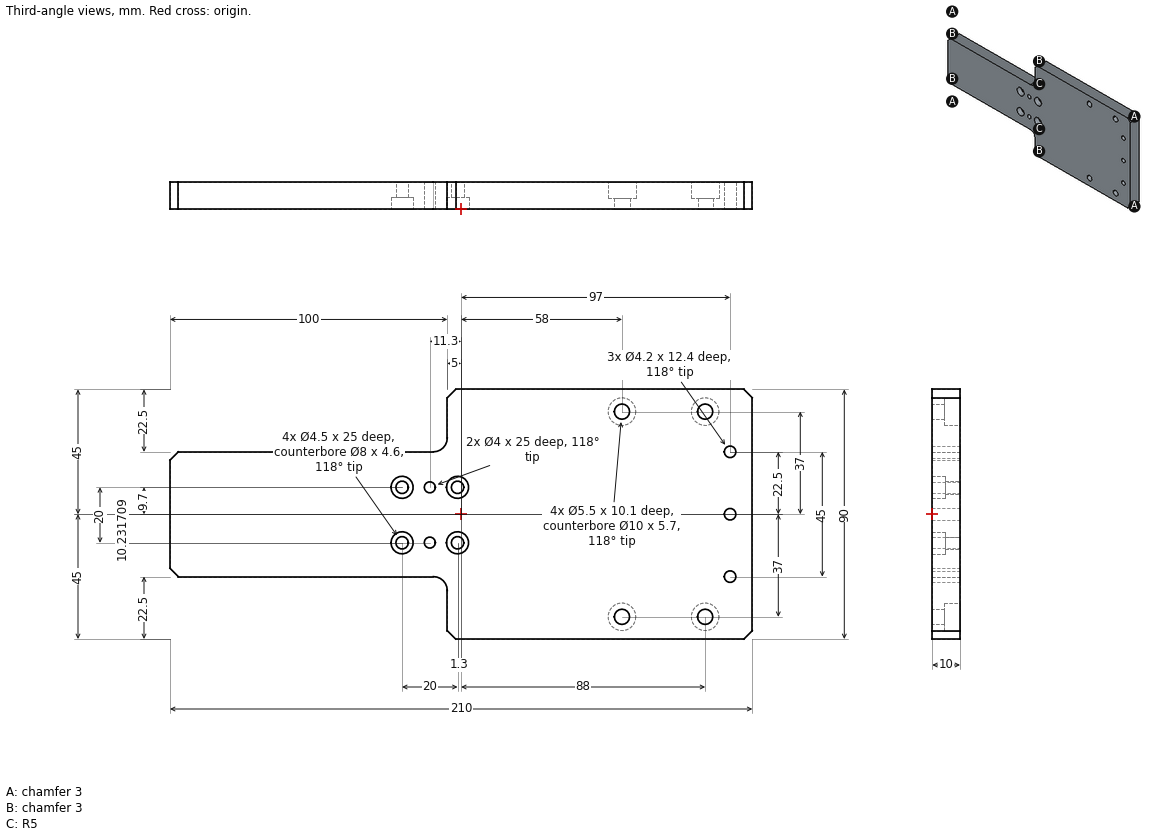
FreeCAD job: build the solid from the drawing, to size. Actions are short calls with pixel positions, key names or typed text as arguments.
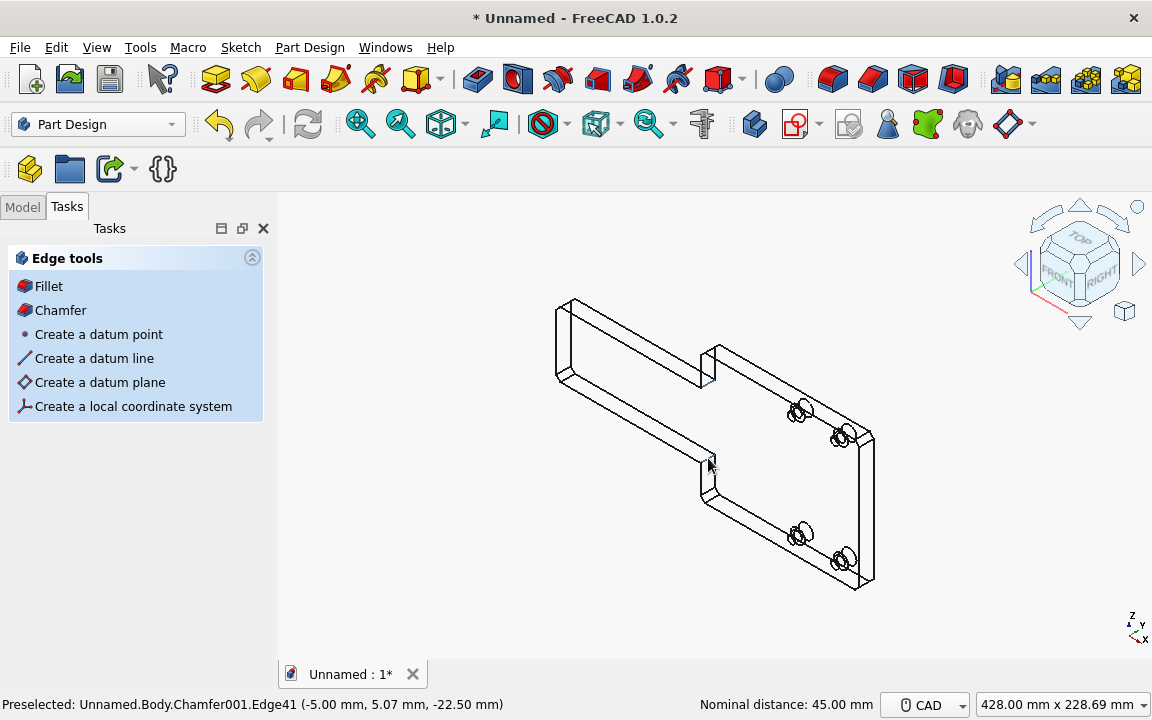
click(834, 80)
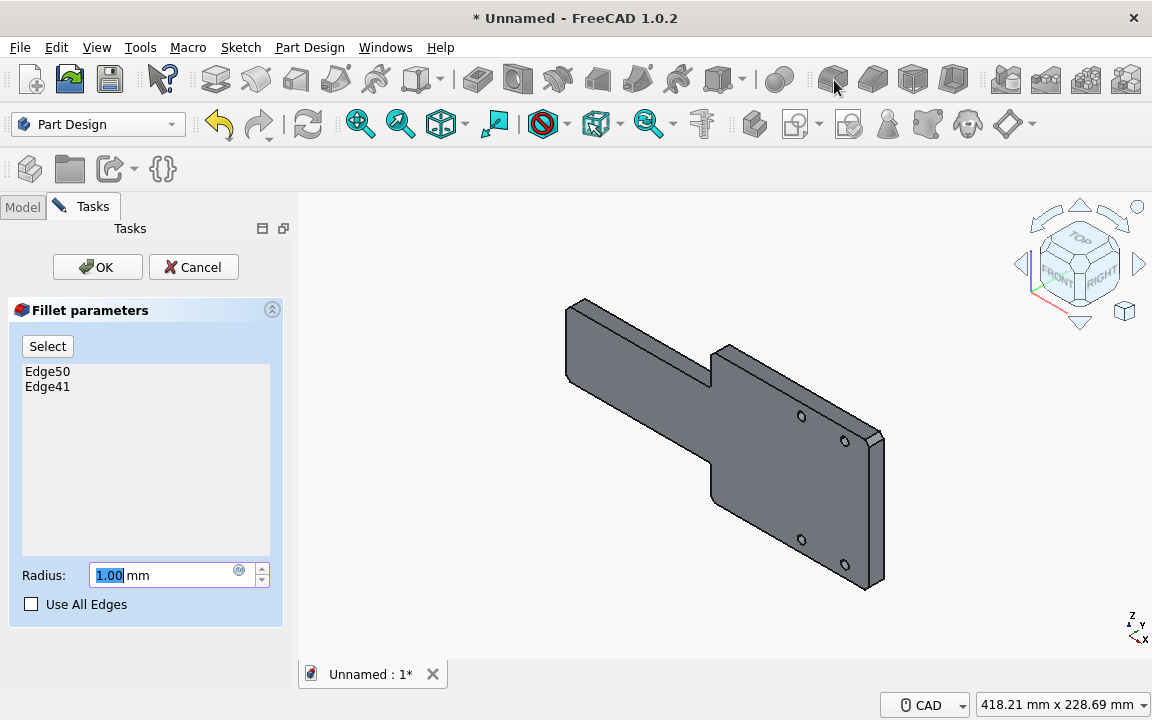
text(5)
key(Tab)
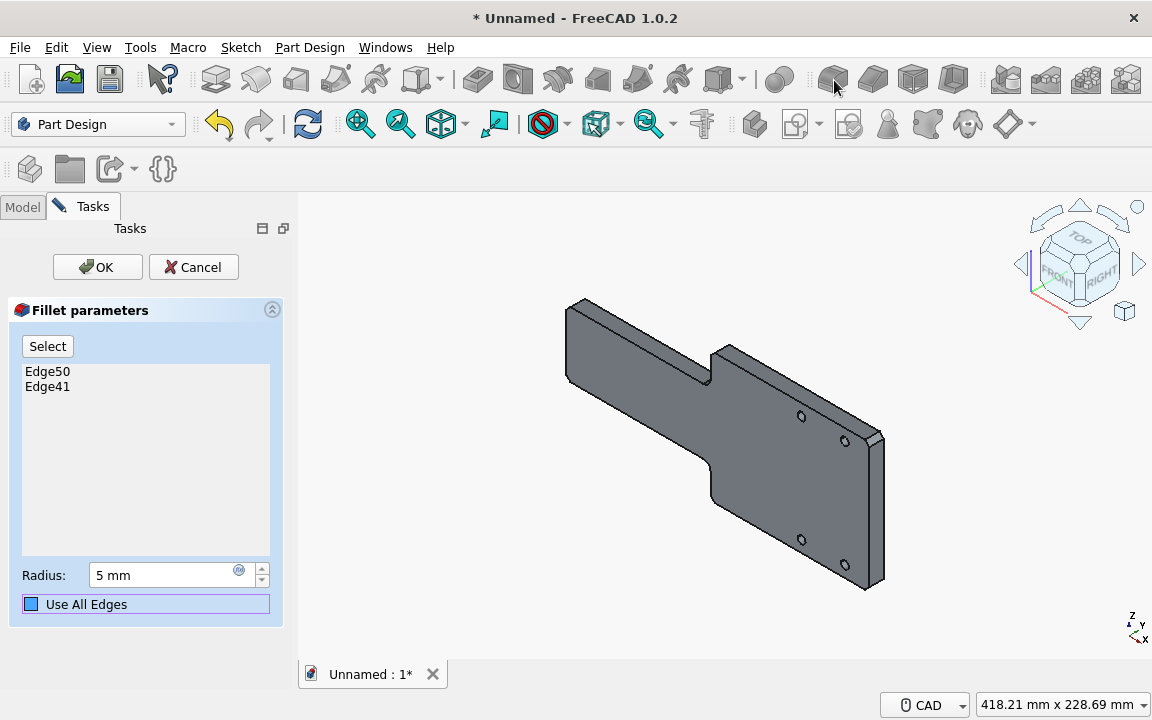
click(98, 267)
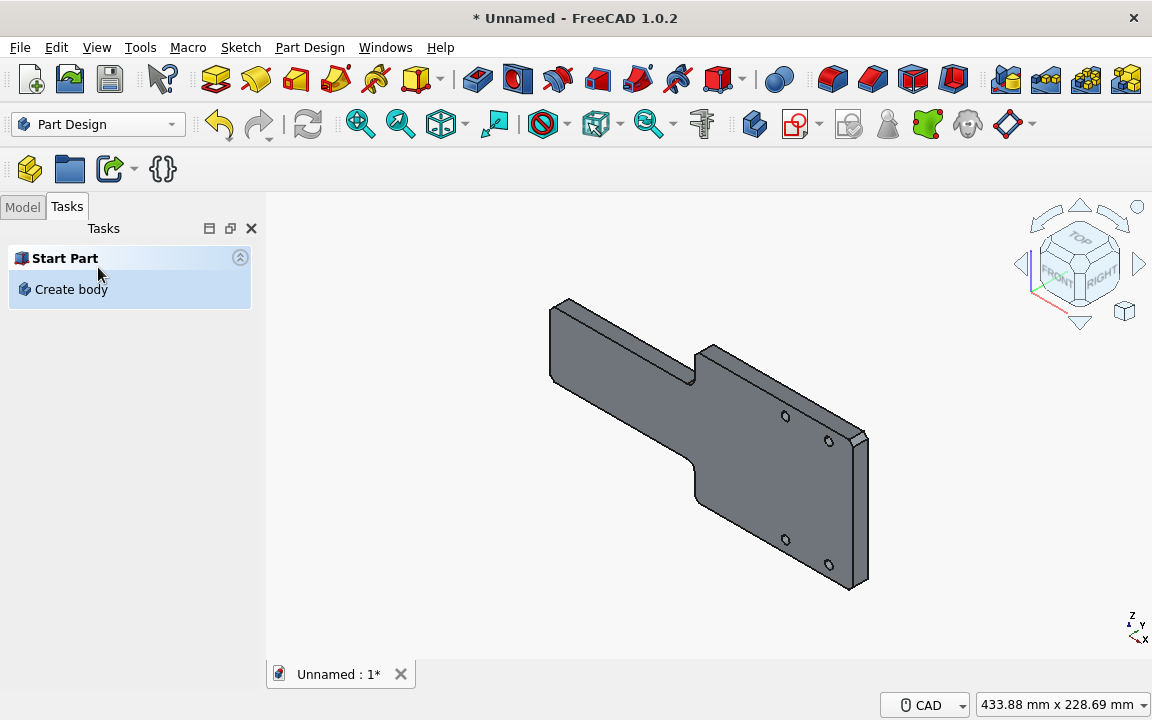
click(796, 124)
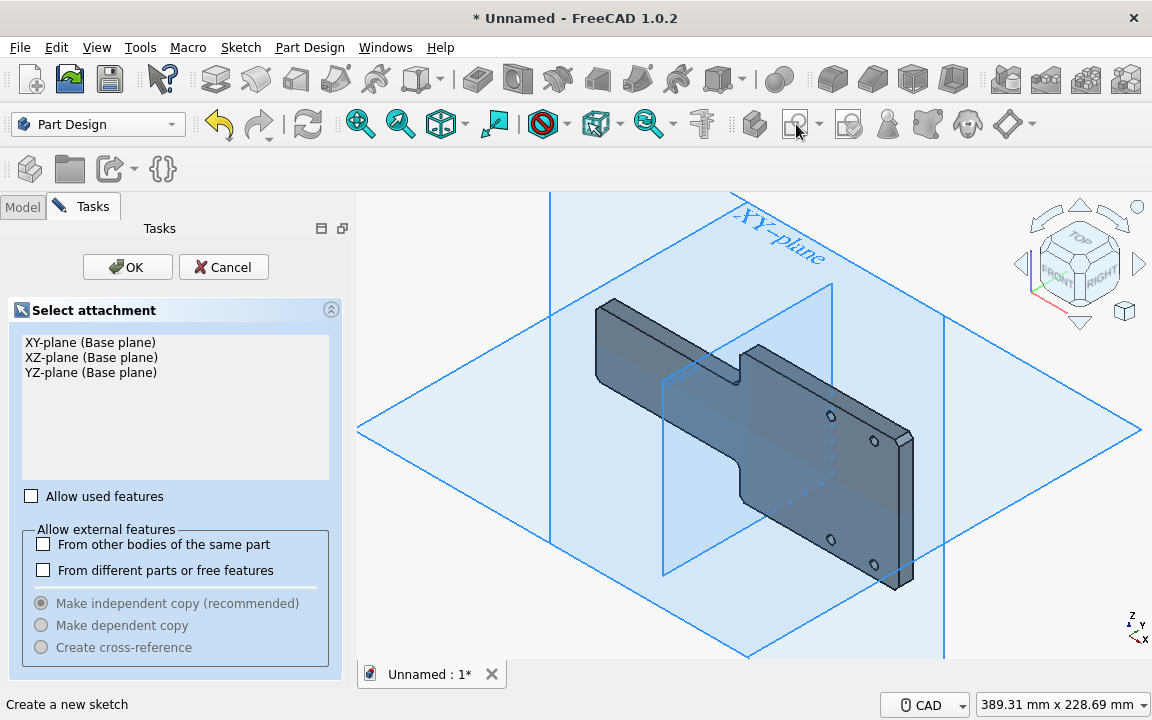
click(82, 358)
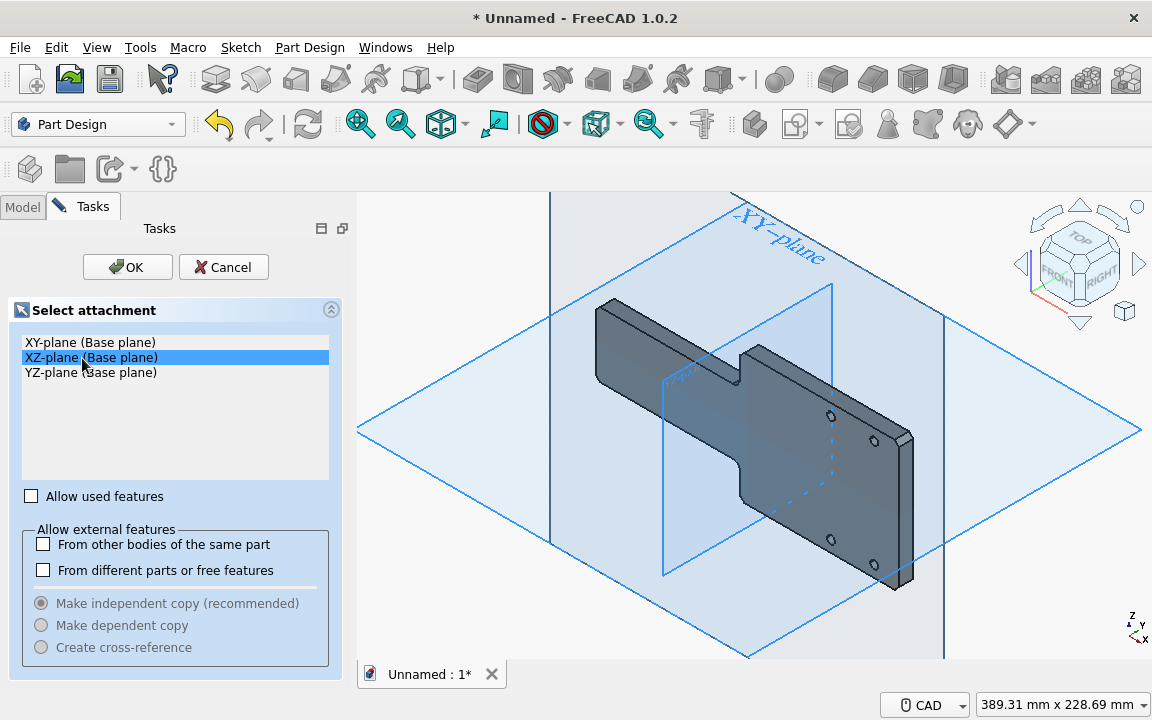
click(128, 267)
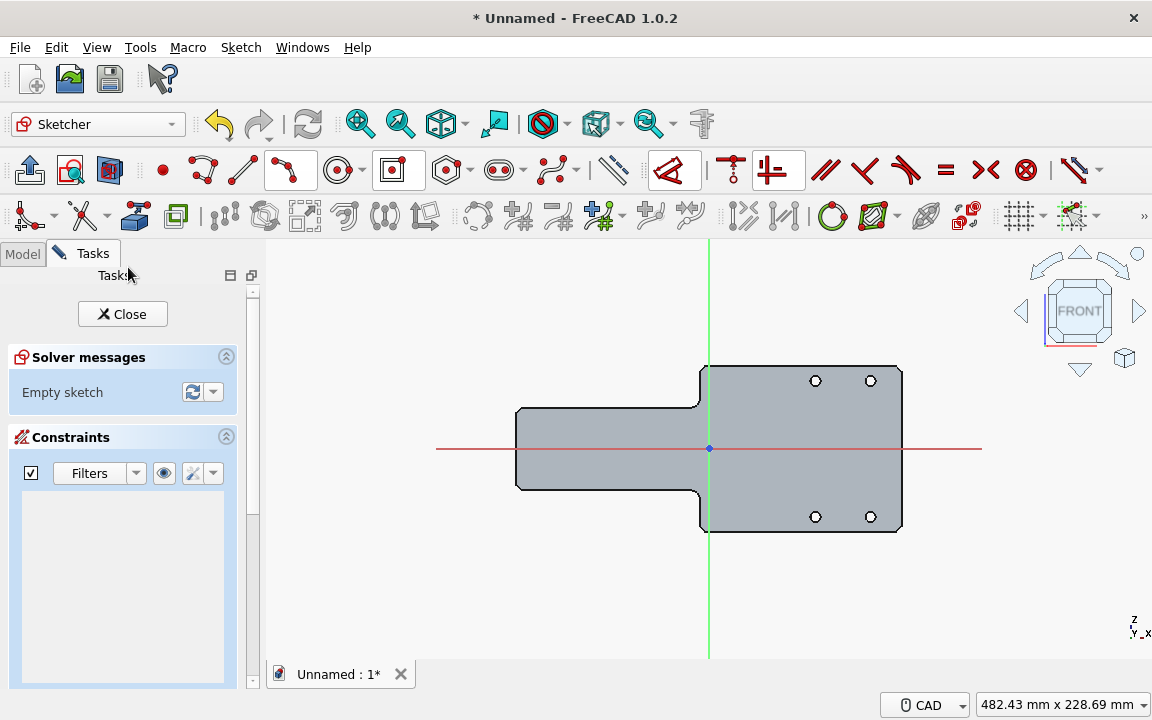
scroll(698, 450, up, 9)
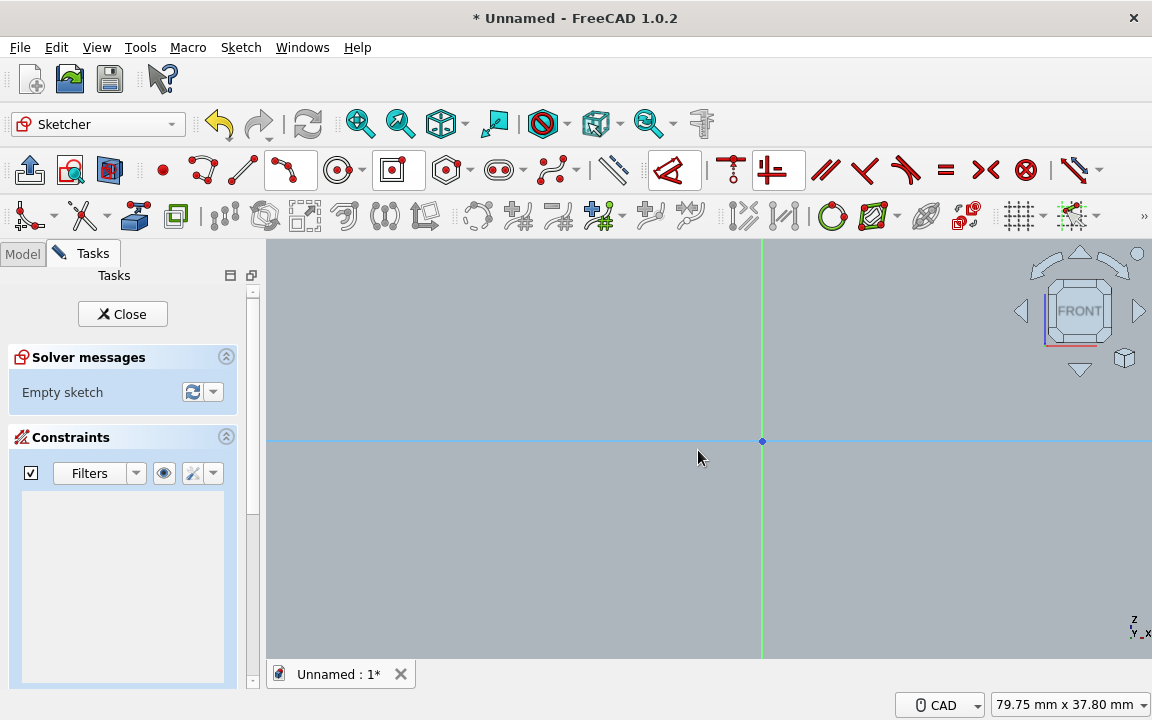
click(338, 170)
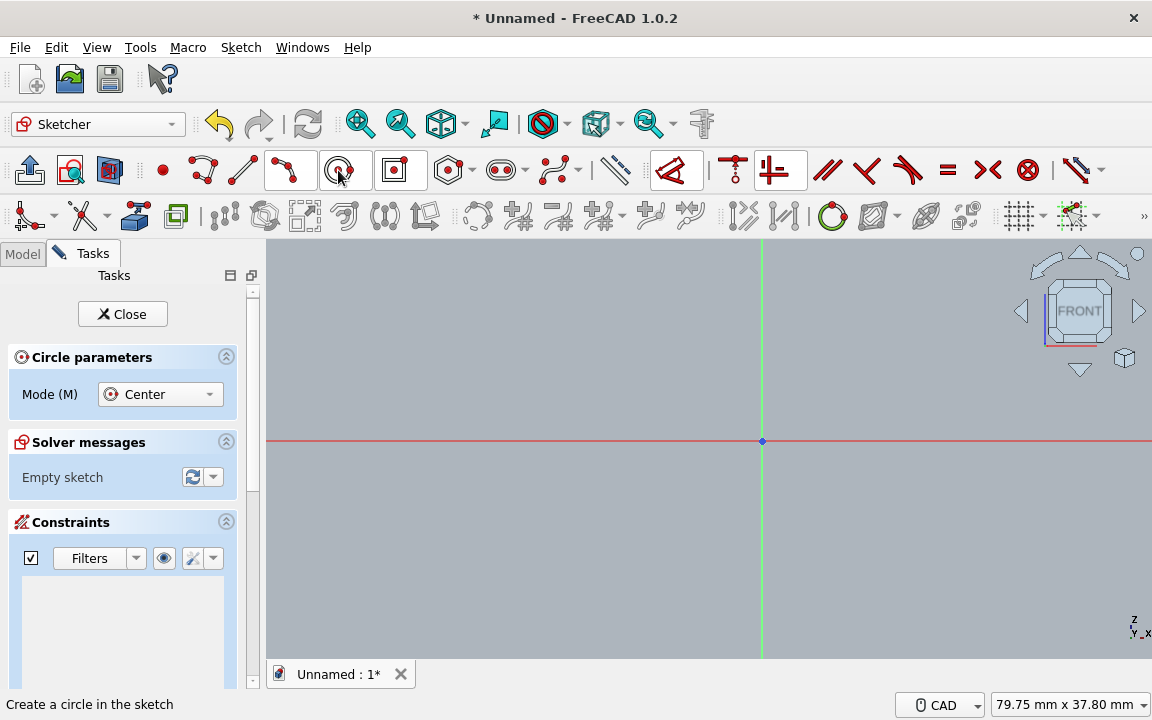
click(525, 556)
click(543, 538)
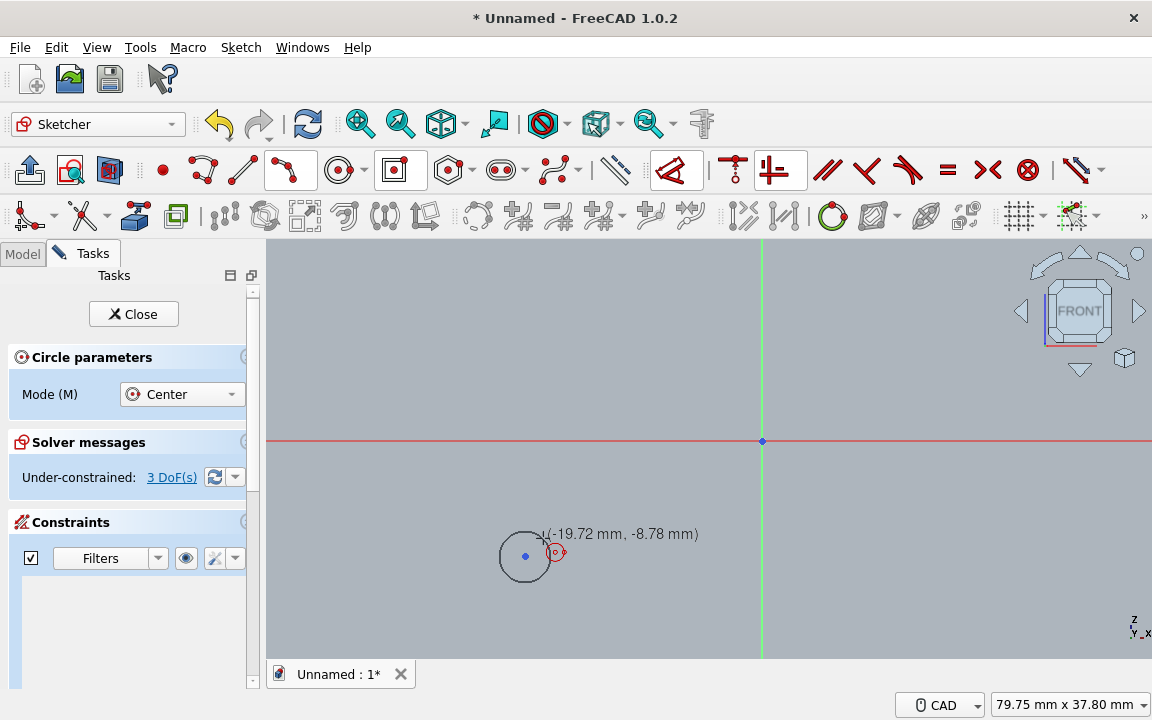
click(525, 334)
click(543, 316)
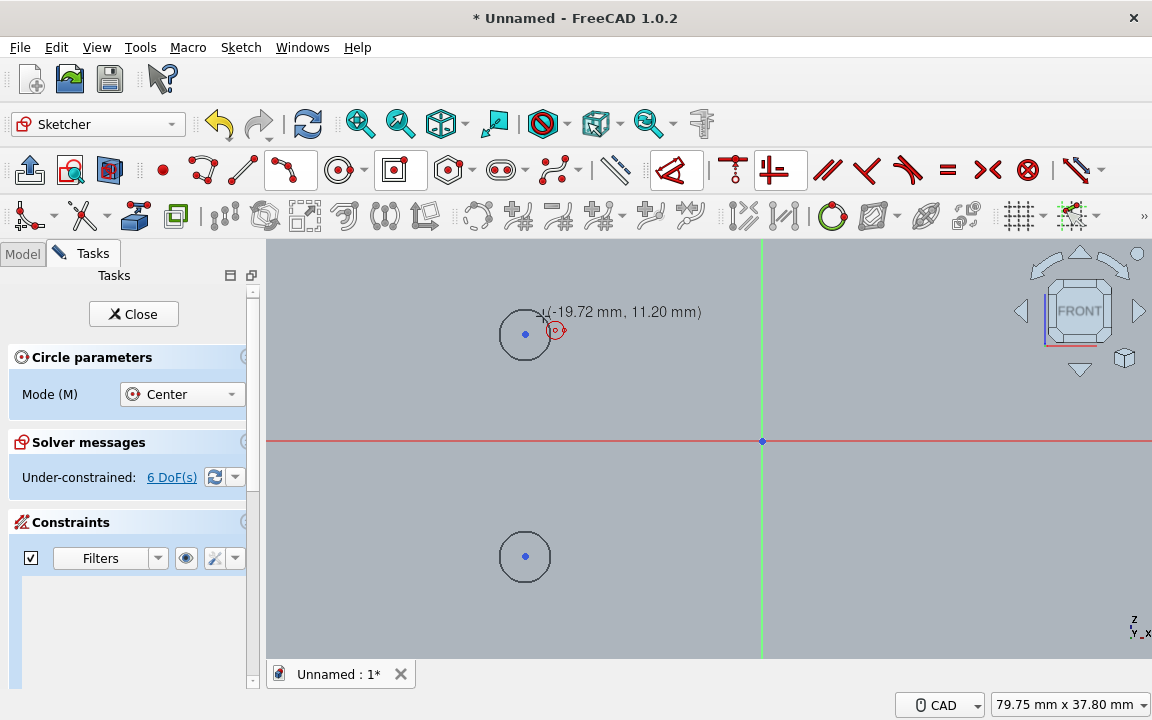
click(748, 556)
click(730, 538)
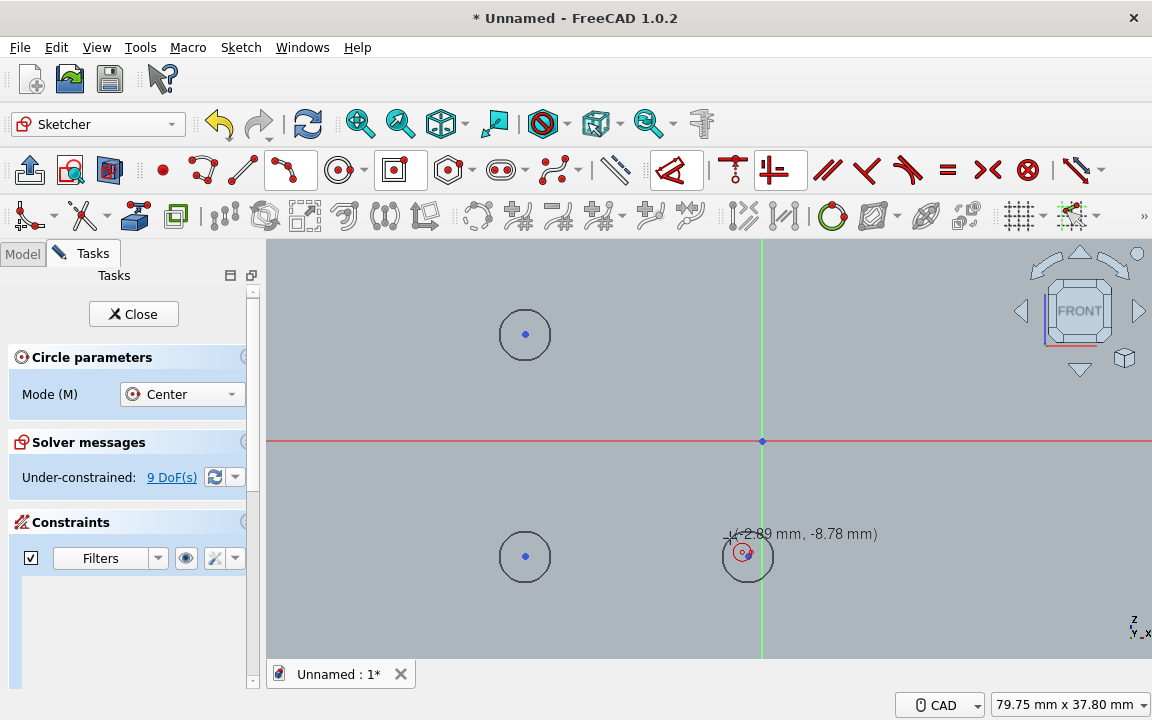
click(748, 334)
click(730, 316)
key(Escape)